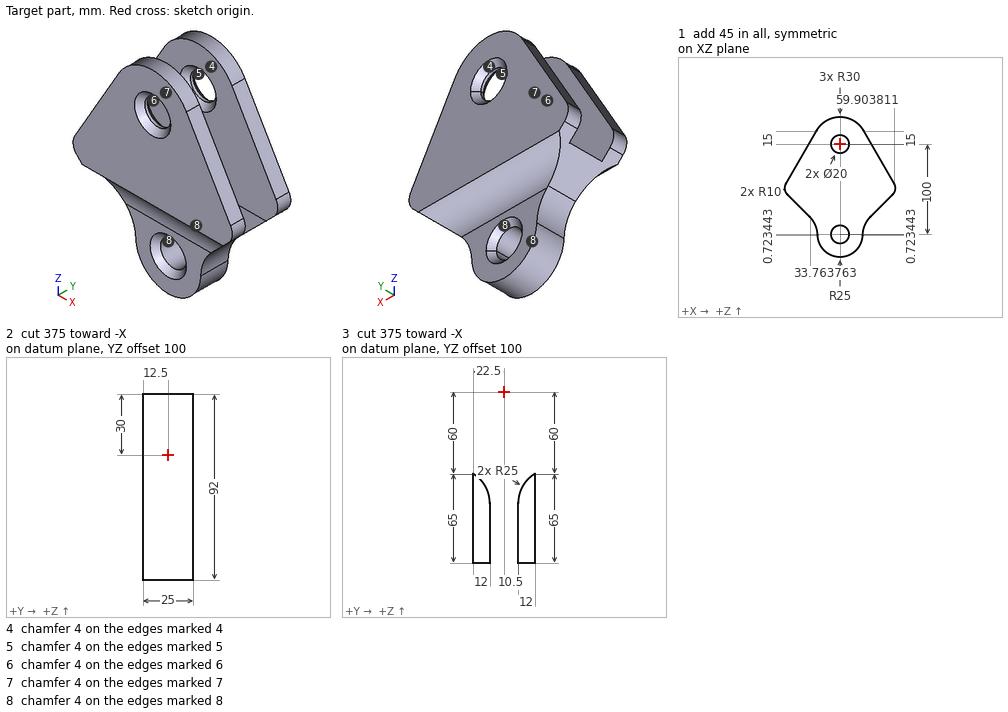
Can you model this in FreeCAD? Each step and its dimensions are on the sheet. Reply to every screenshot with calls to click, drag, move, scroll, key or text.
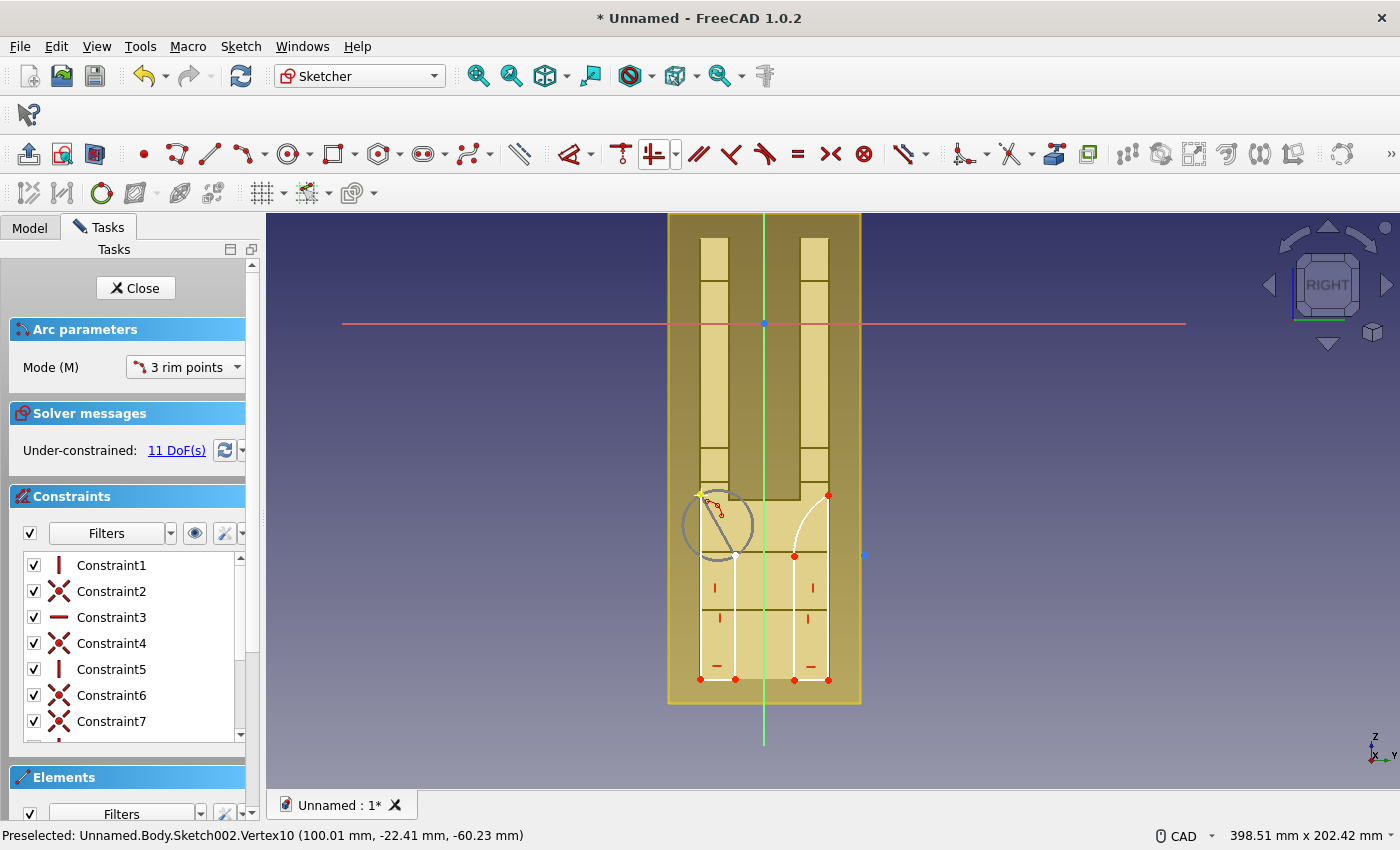
scroll(725, 520, up, 3)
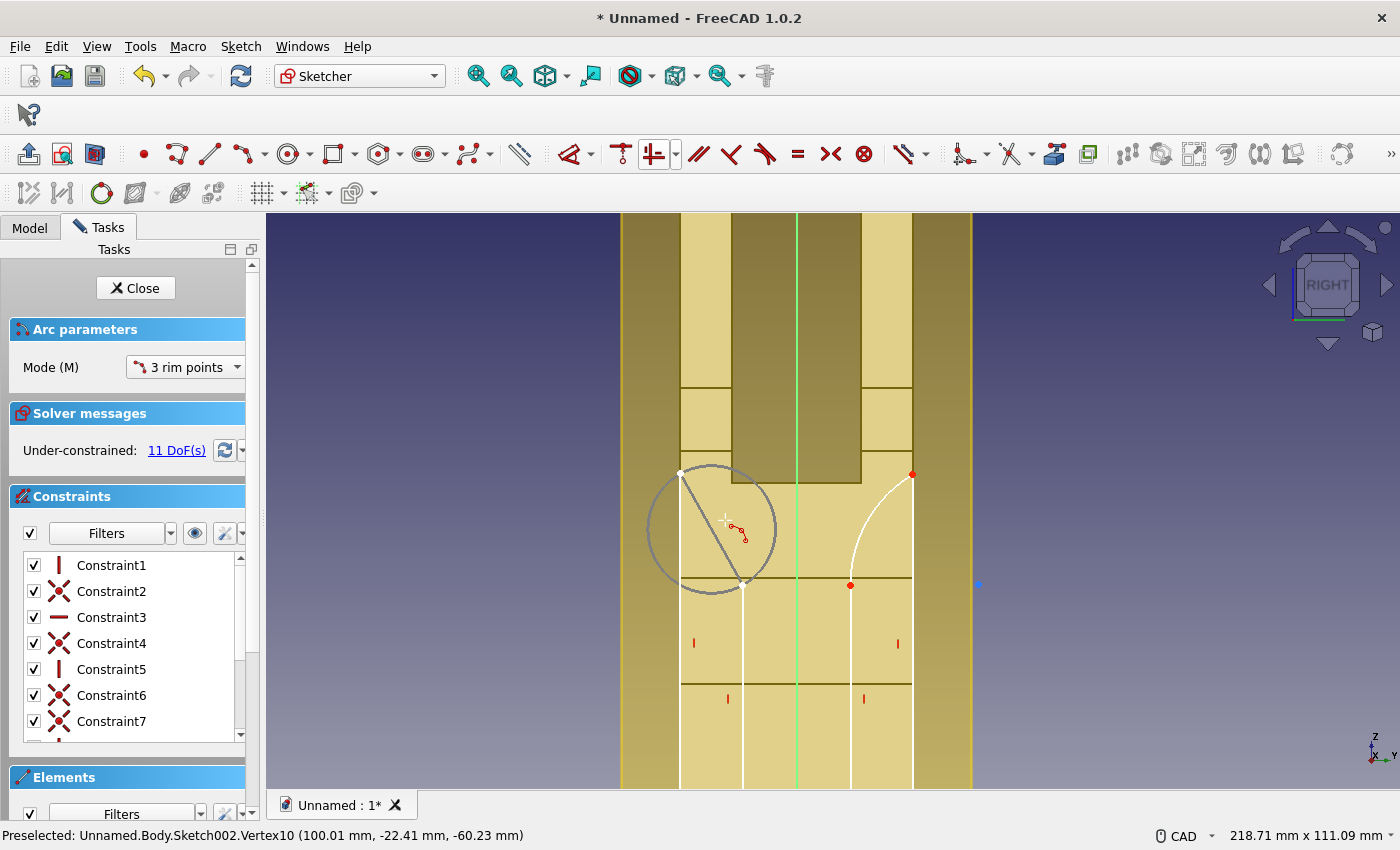
click(726, 520)
key(Escape)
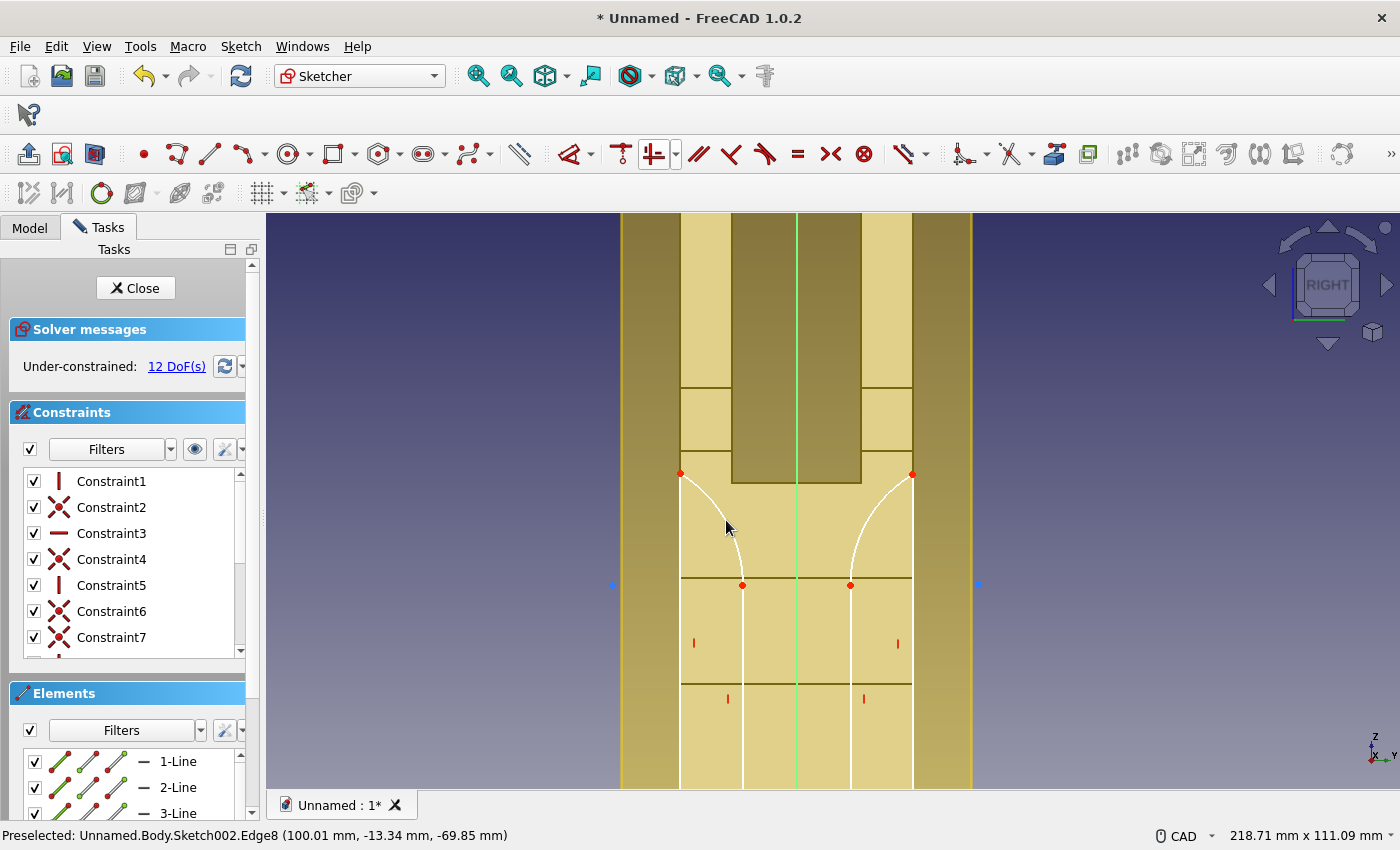
click(851, 654)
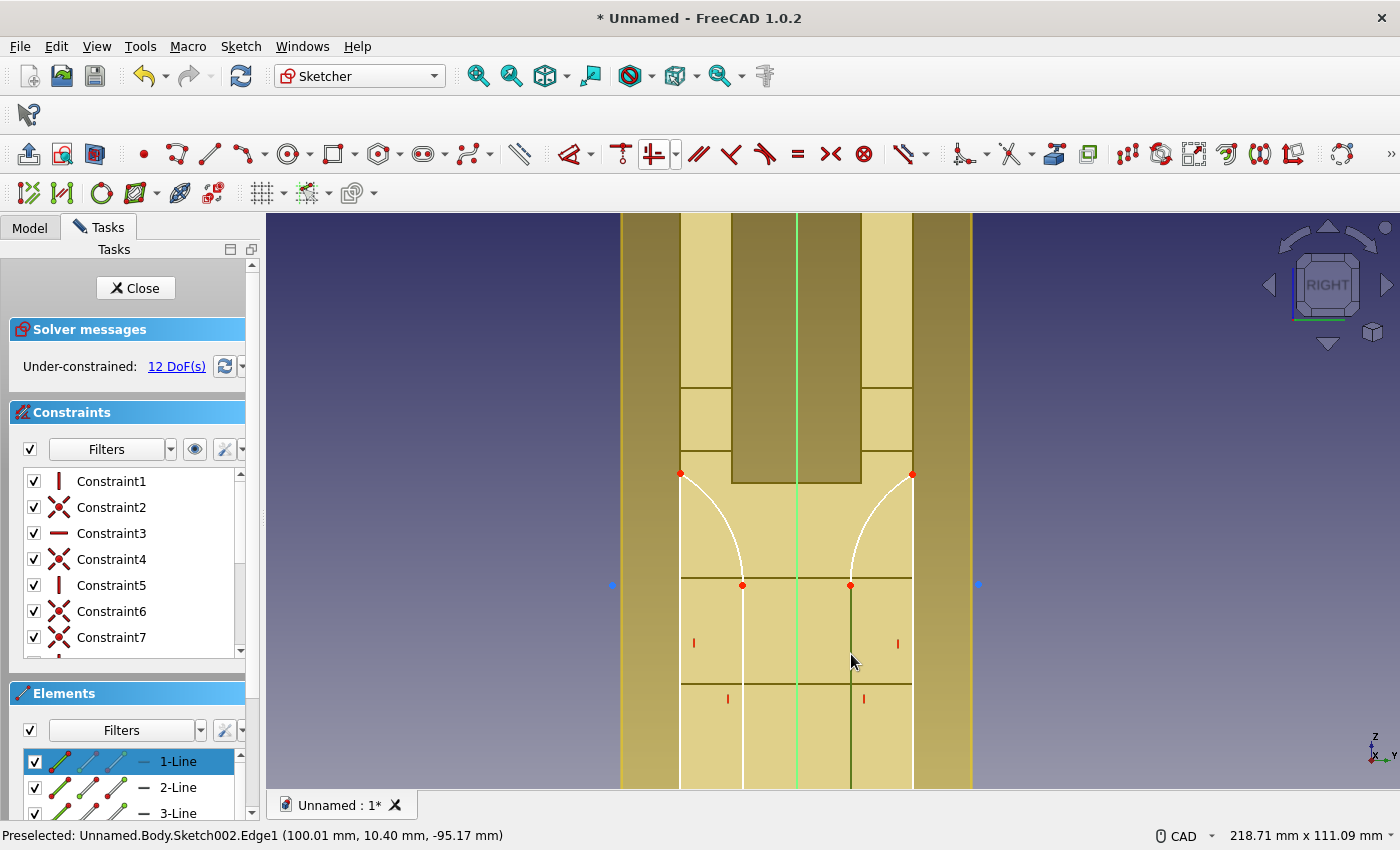
click(882, 500)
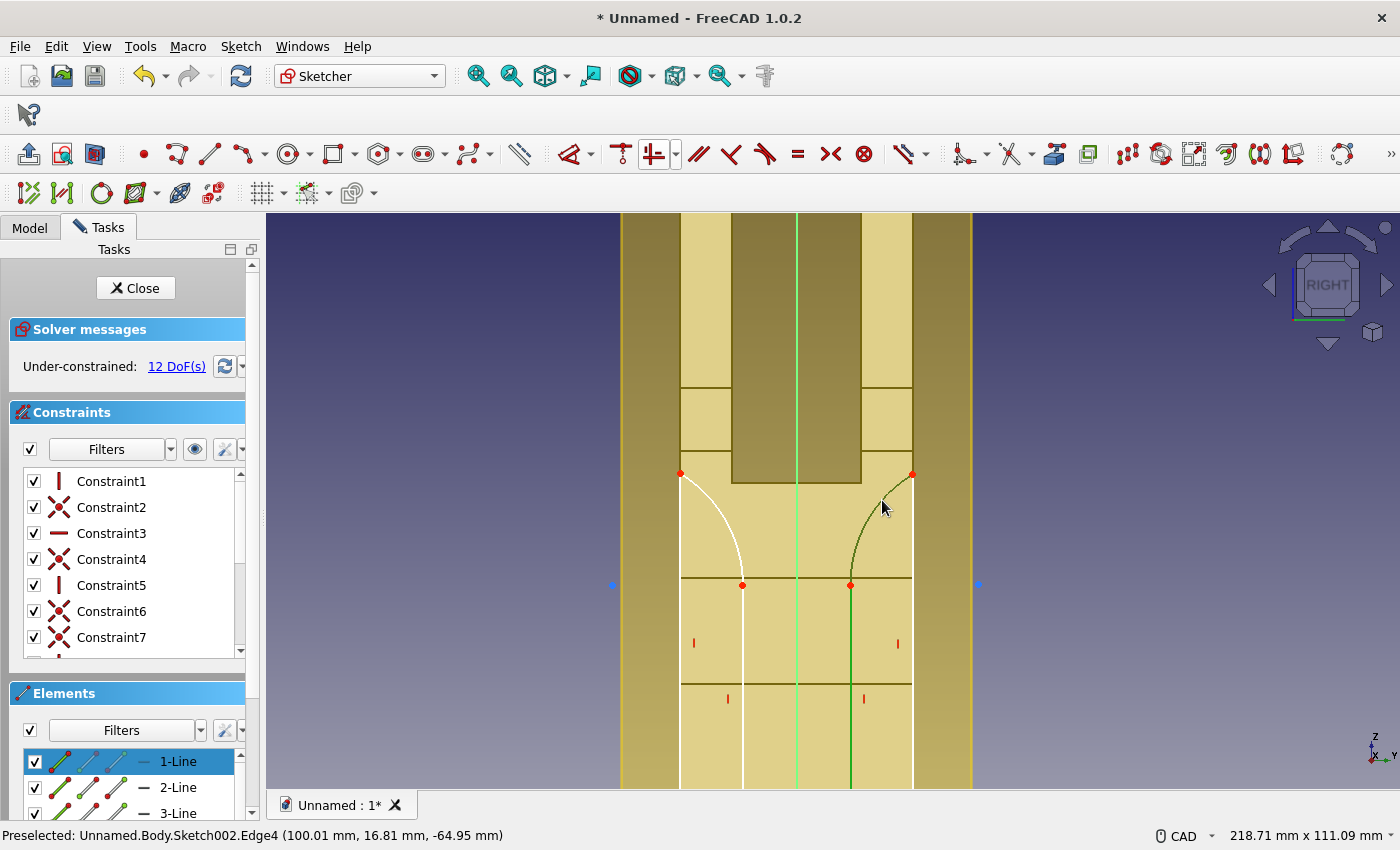
click(765, 154)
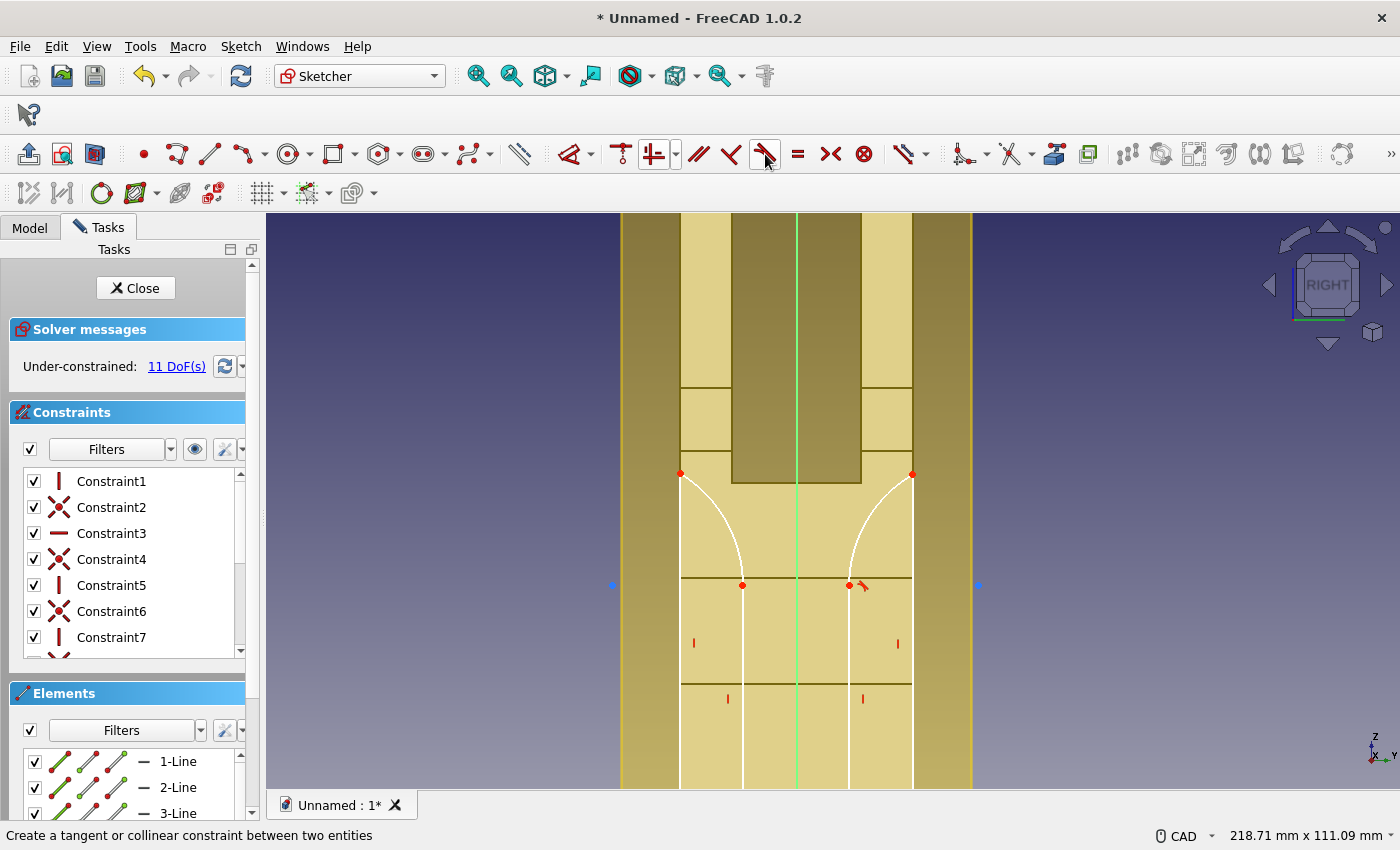
click(743, 743)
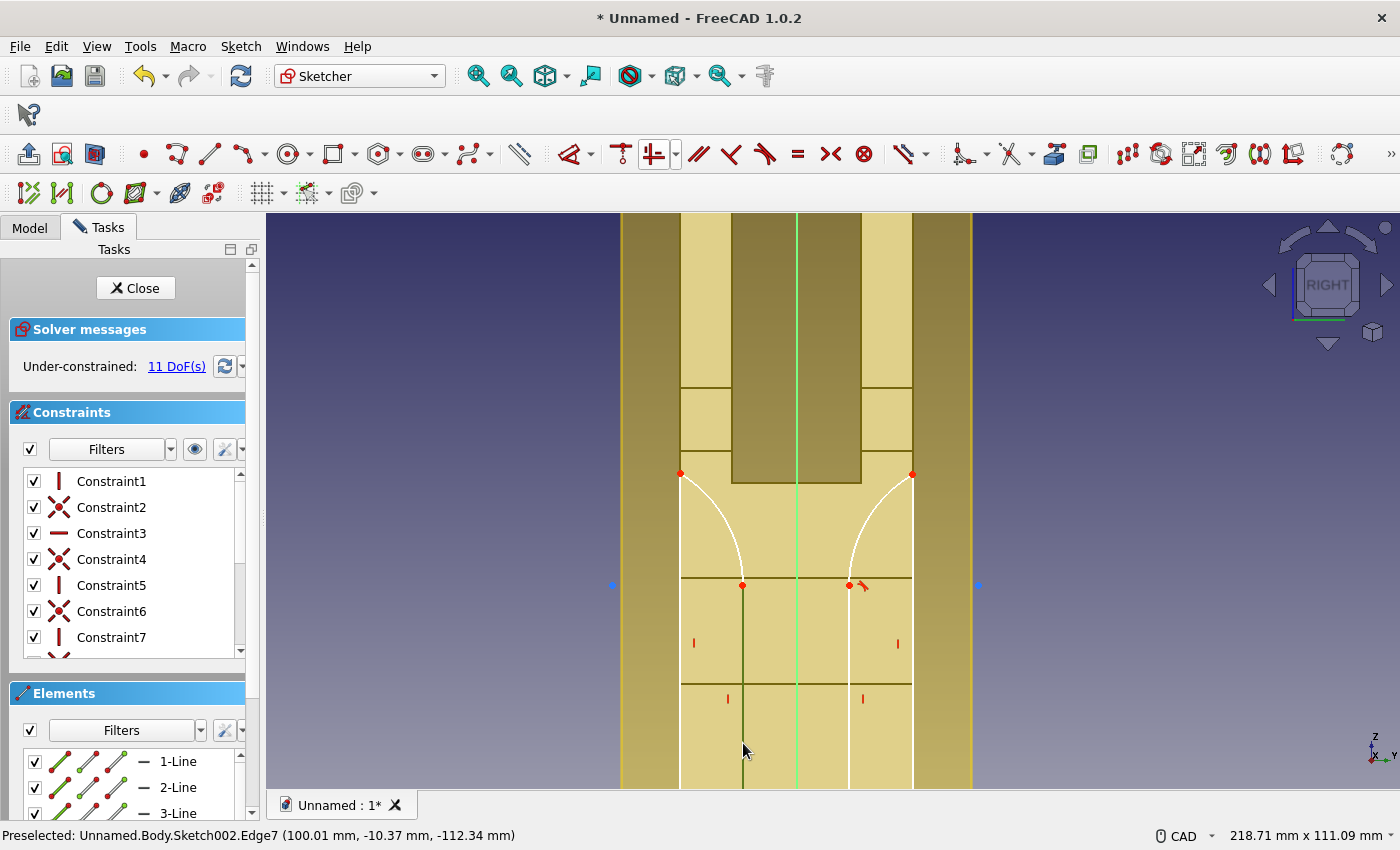
click(737, 546)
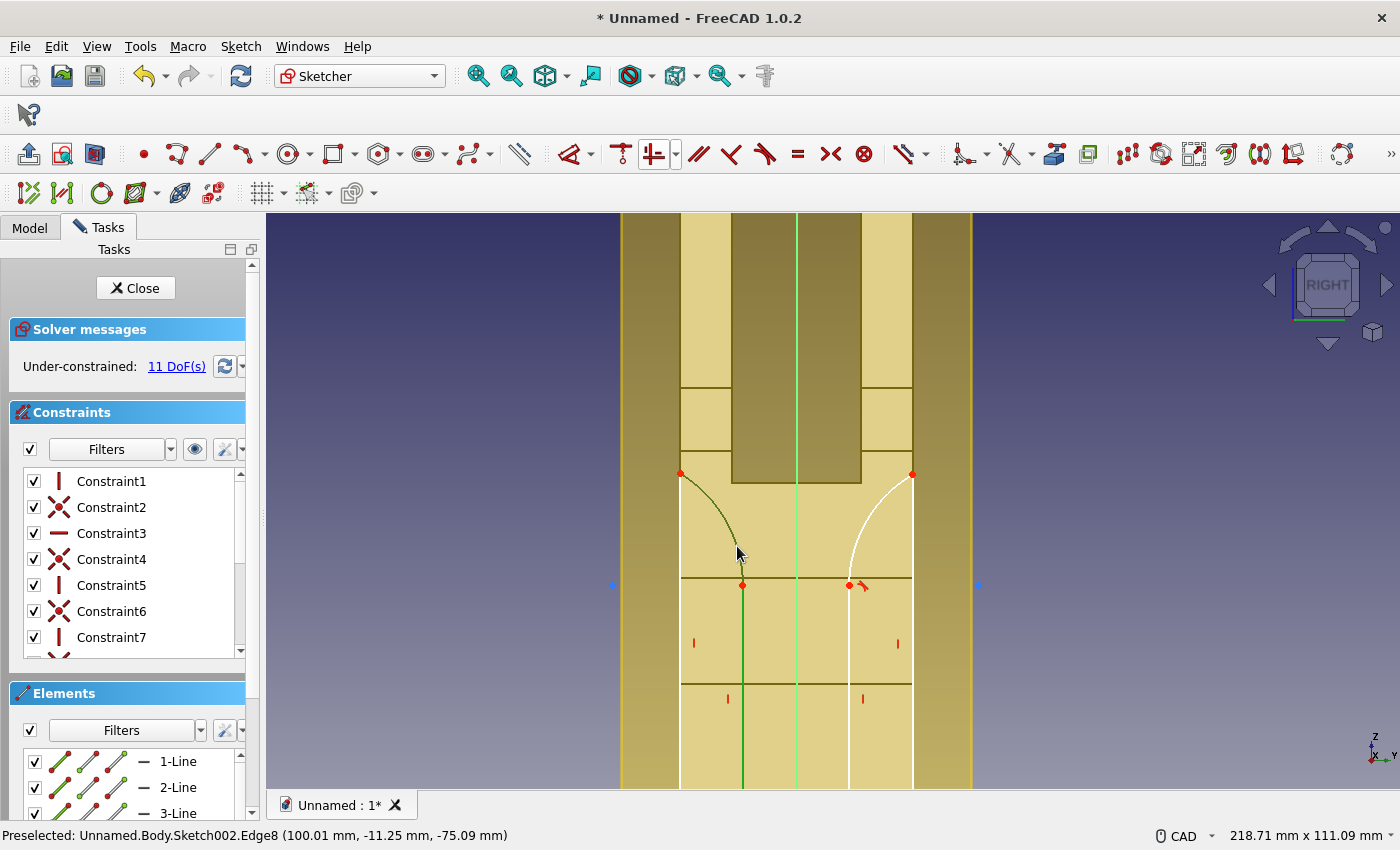
click(765, 154)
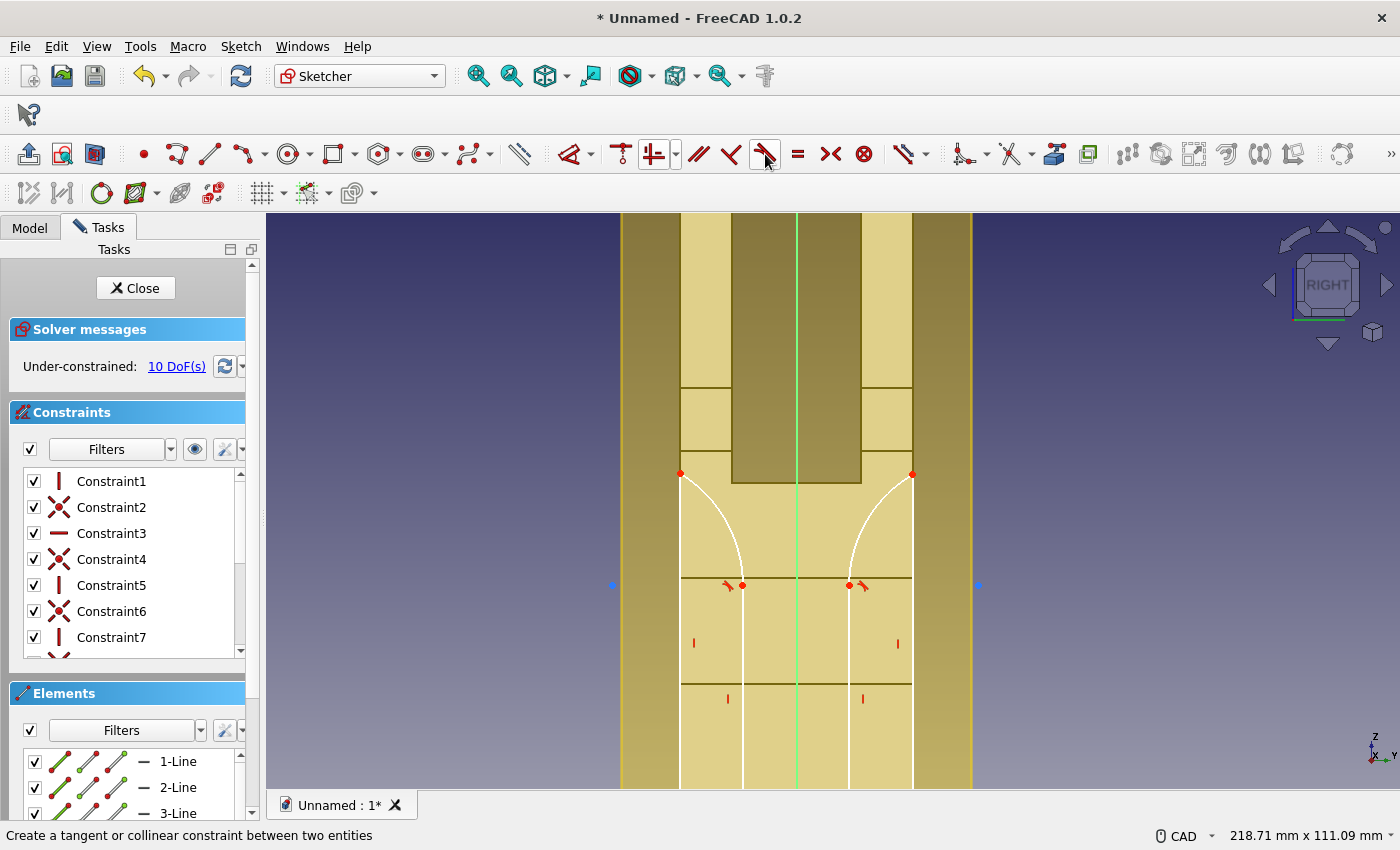
click(882, 500)